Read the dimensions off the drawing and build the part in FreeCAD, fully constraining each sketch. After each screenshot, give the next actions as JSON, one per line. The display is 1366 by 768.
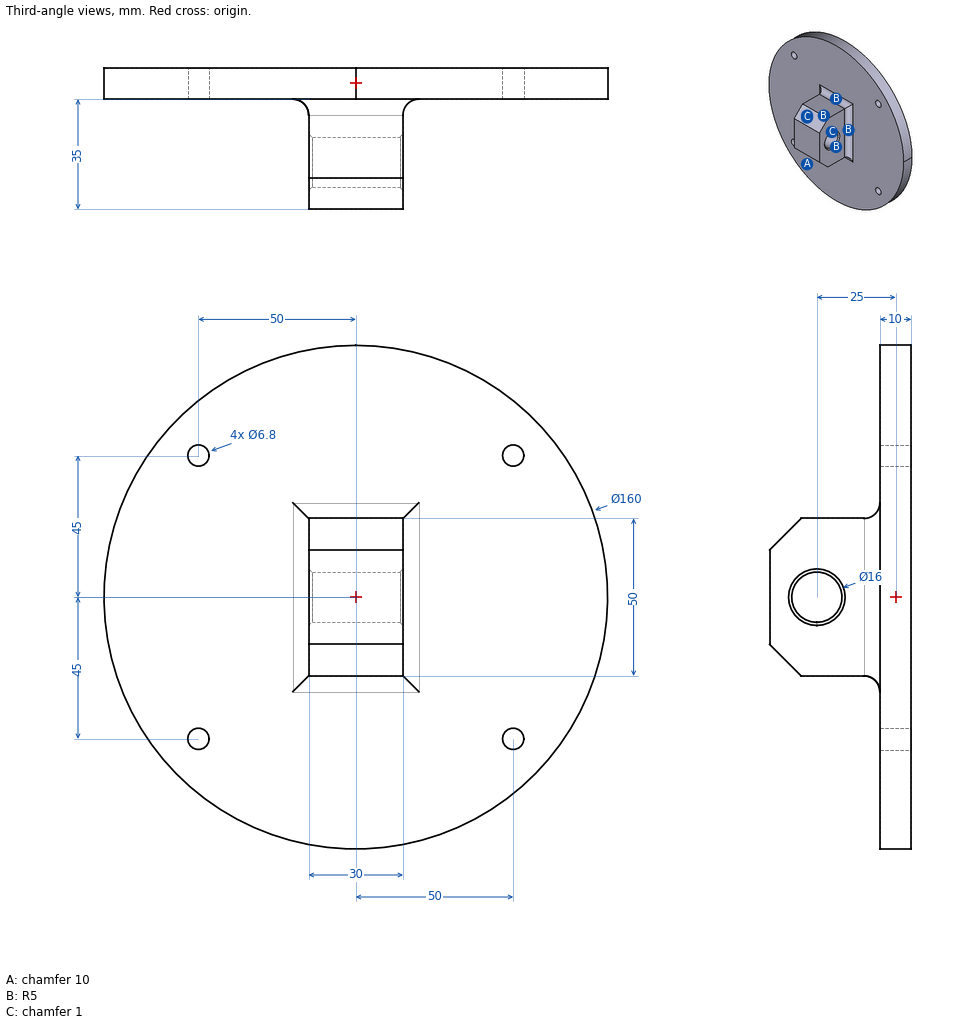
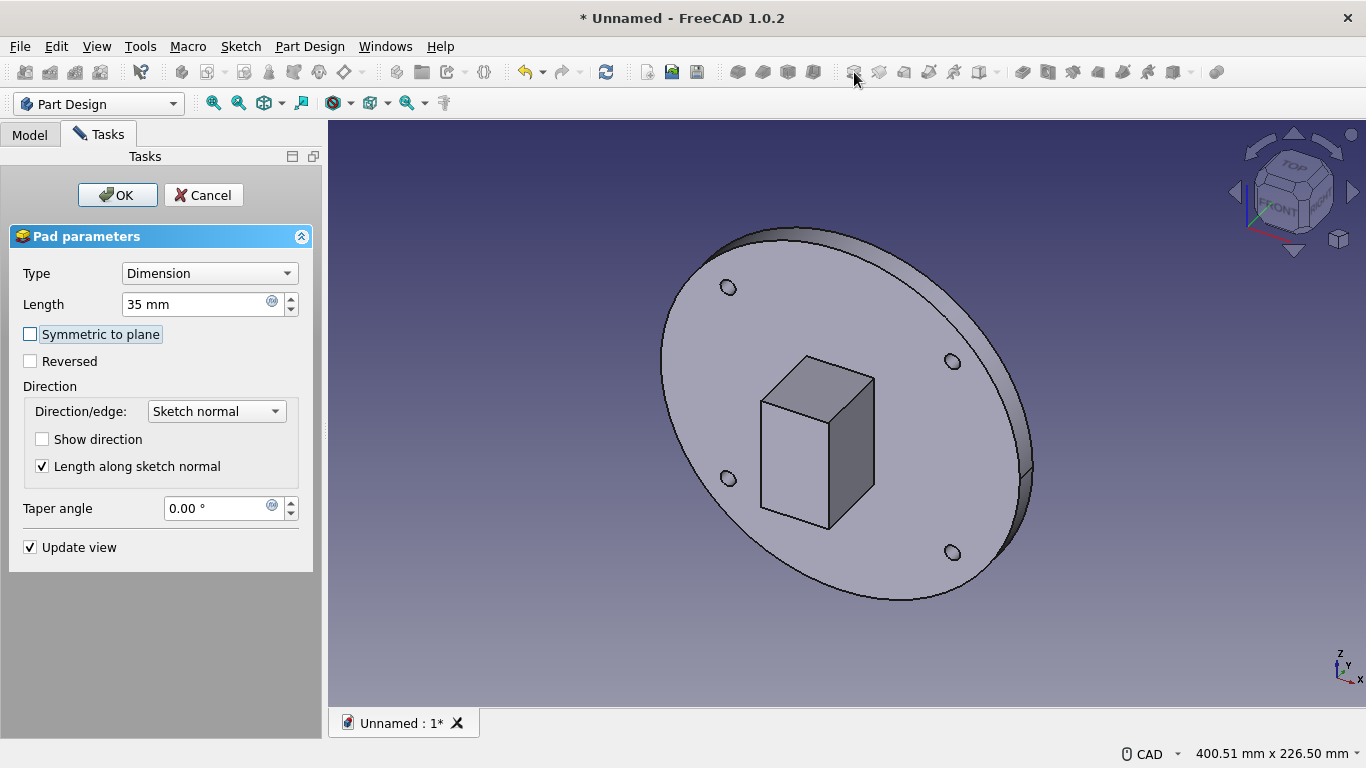
{"action": "left_click", "coordinate": [118, 195]}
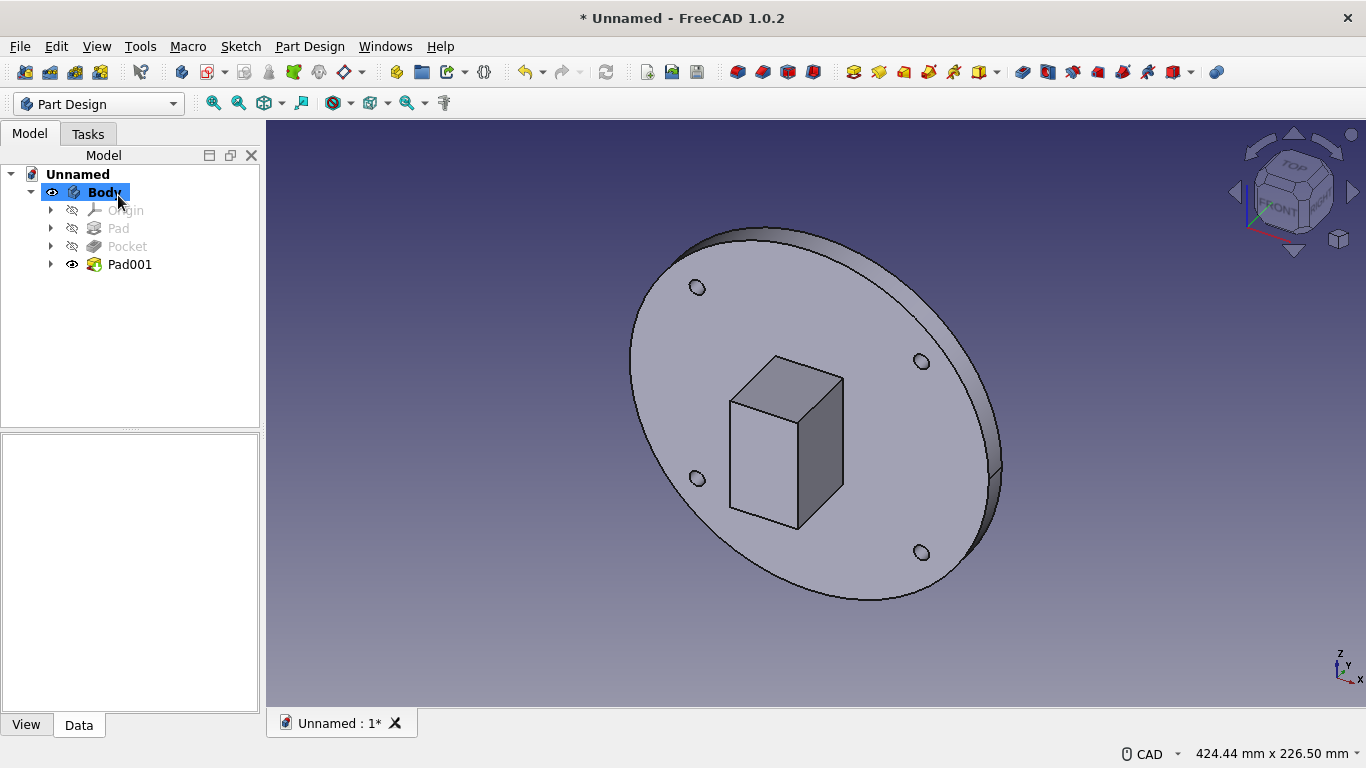
{"action": "left_click", "coordinate": [820, 438]}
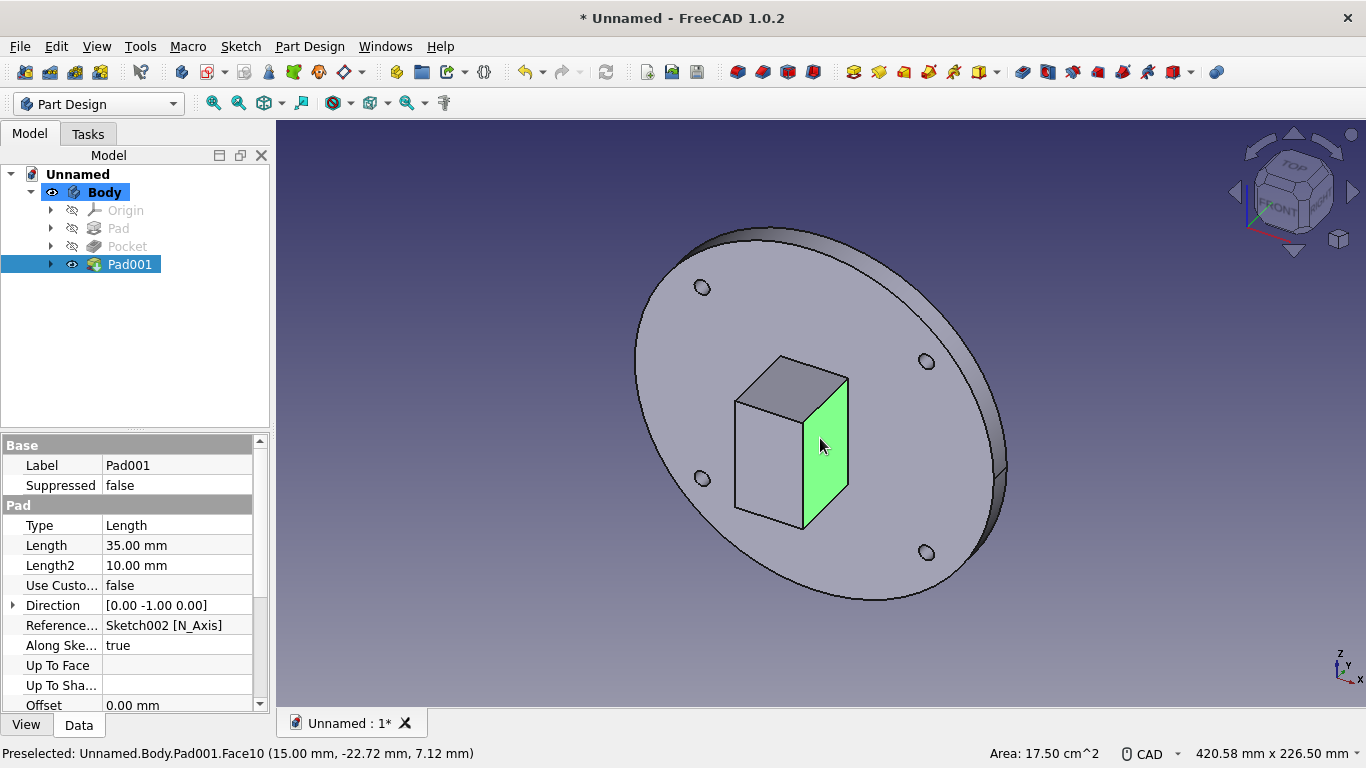
{"action": "left_click", "coordinate": [206, 72]}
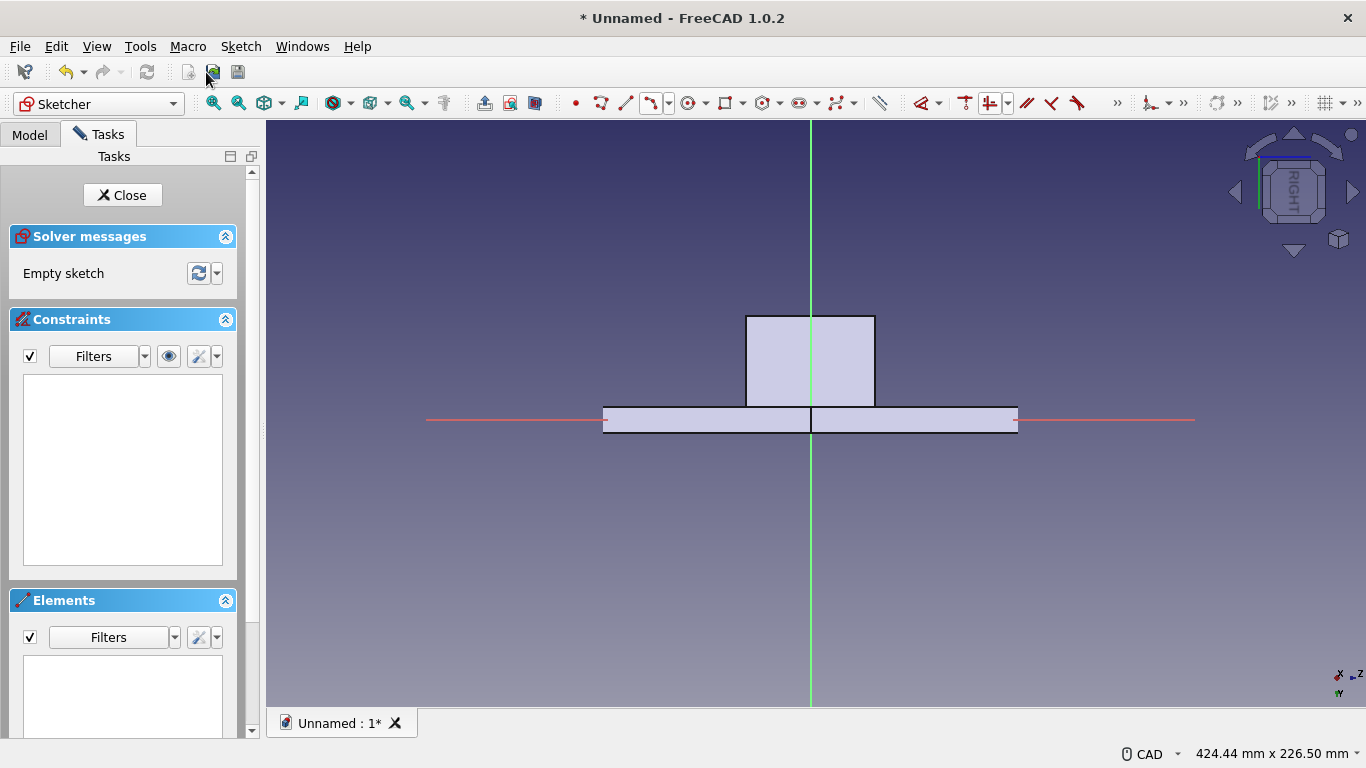
{"action": "left_click", "coordinate": [535, 104]}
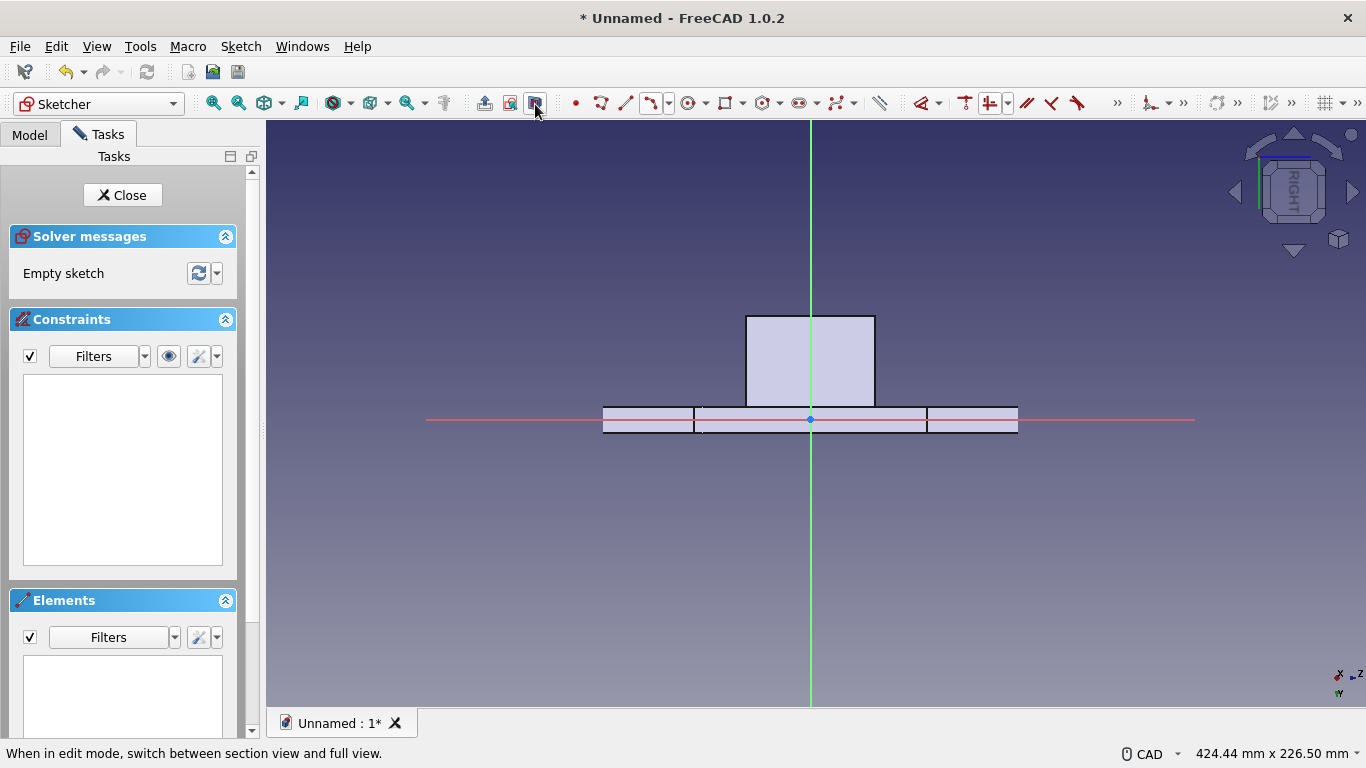
{"action": "scroll", "coordinate": [831, 365], "scroll_direction": "up", "scroll_amount": 7}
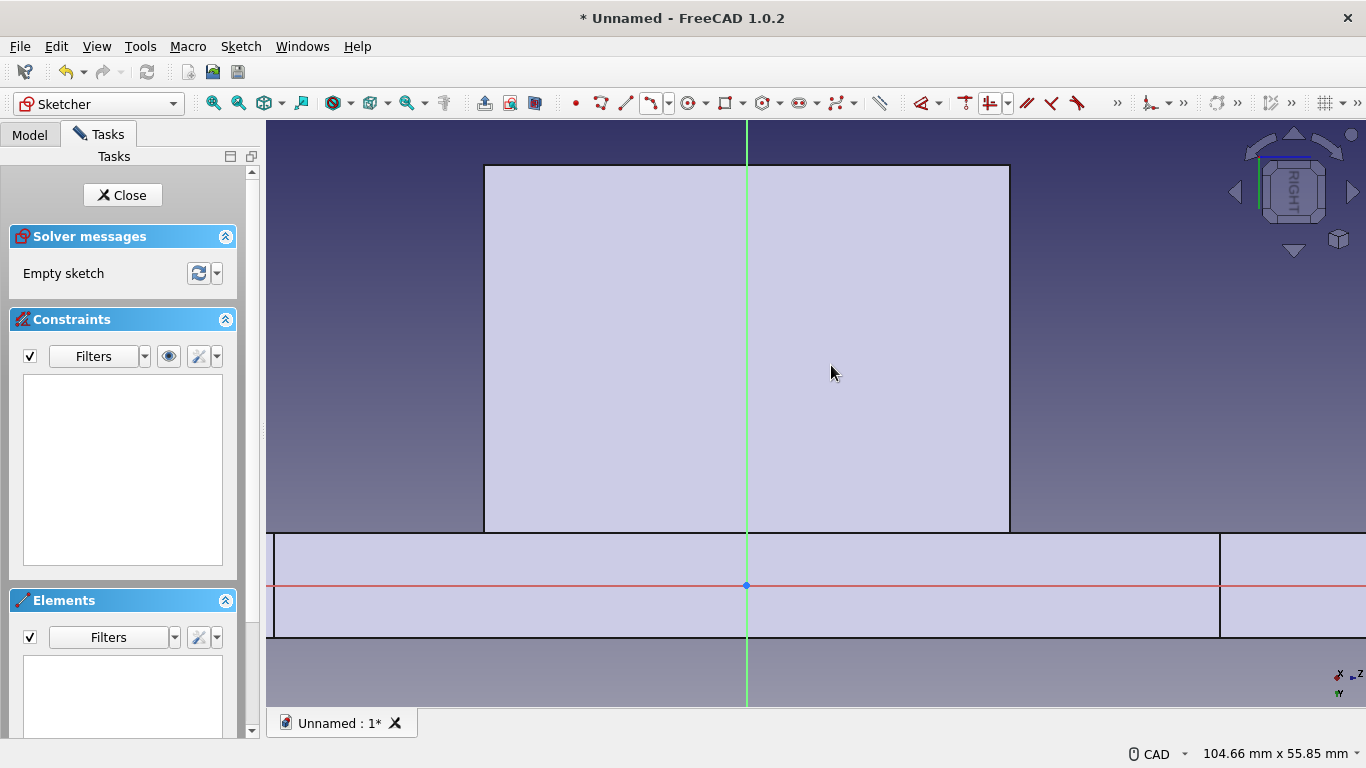
{"action": "key", "text": "g c"}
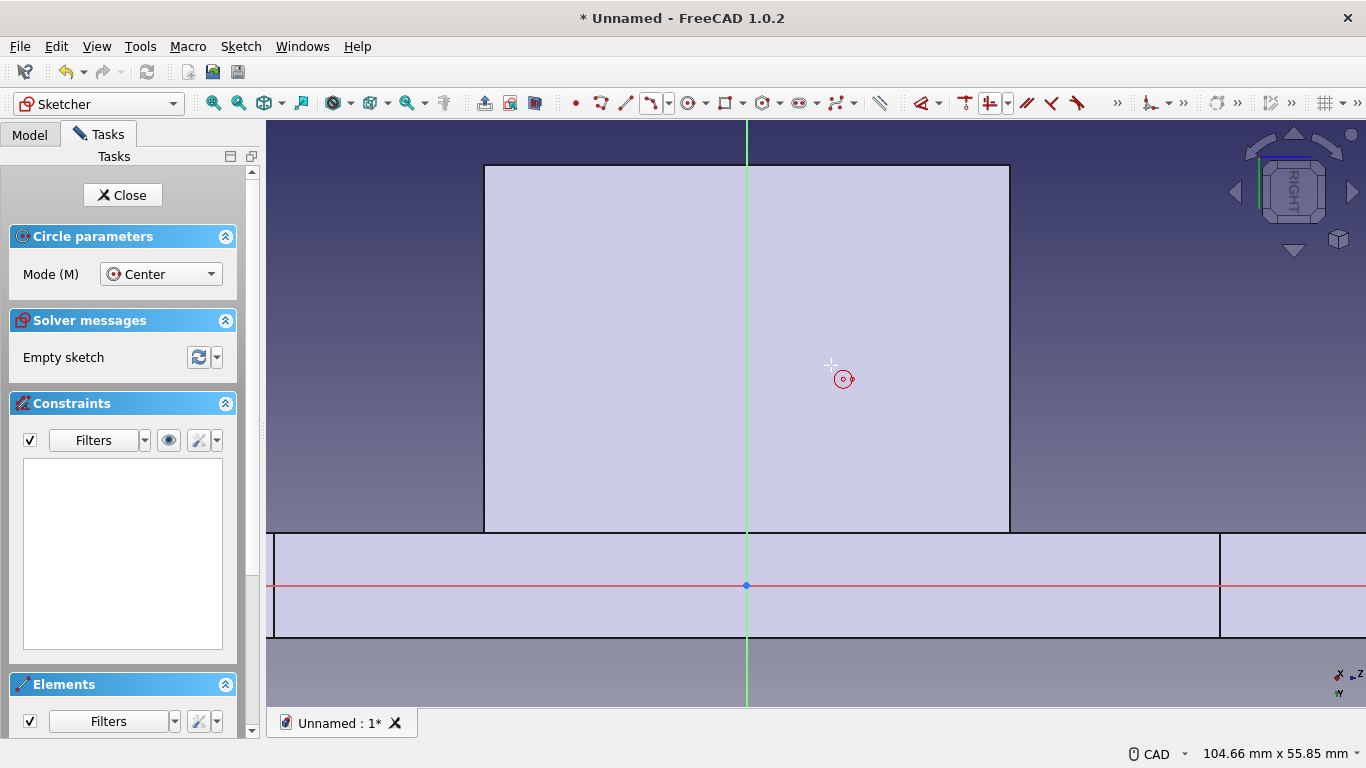
{"action": "left_click", "coordinate": [747, 323]}
{"action": "left_click", "coordinate": [806, 263]}
{"action": "key", "text": "Escape"}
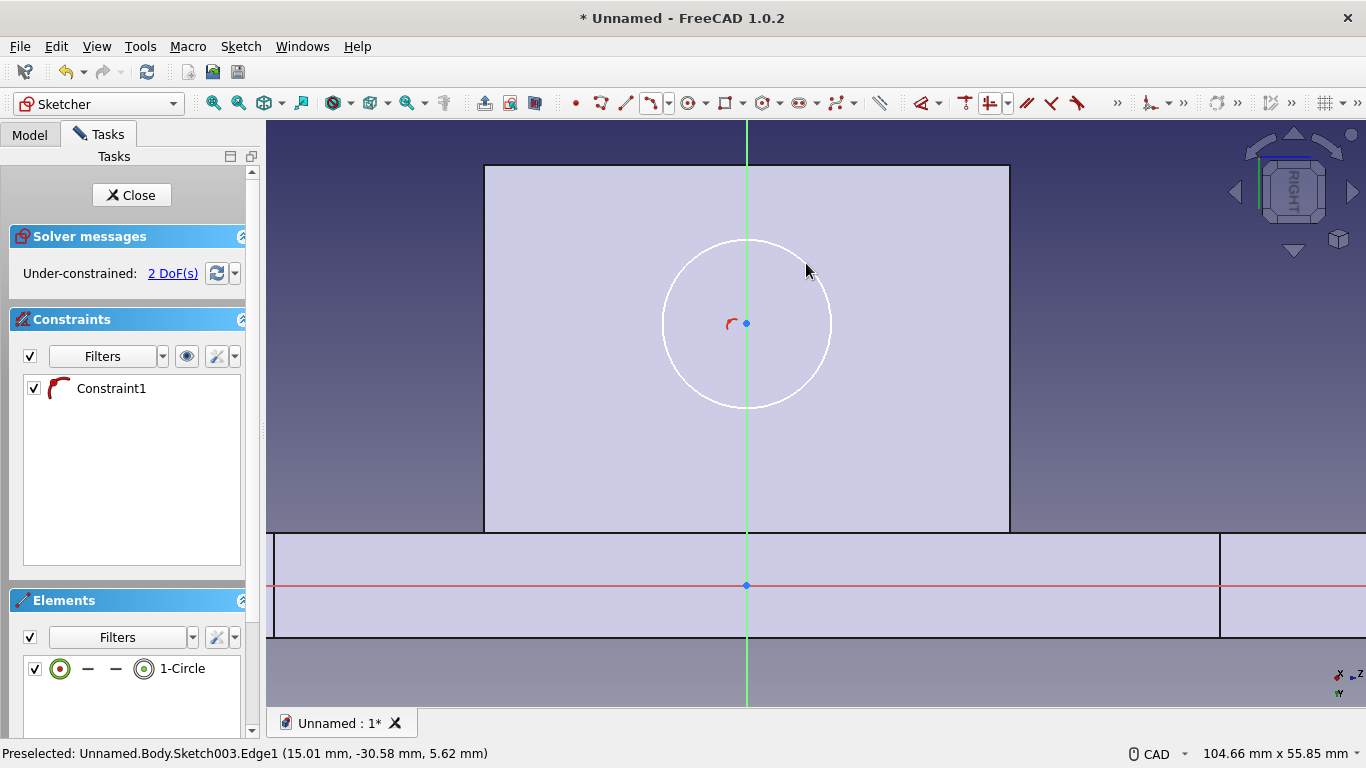
{"action": "key", "text": "d"}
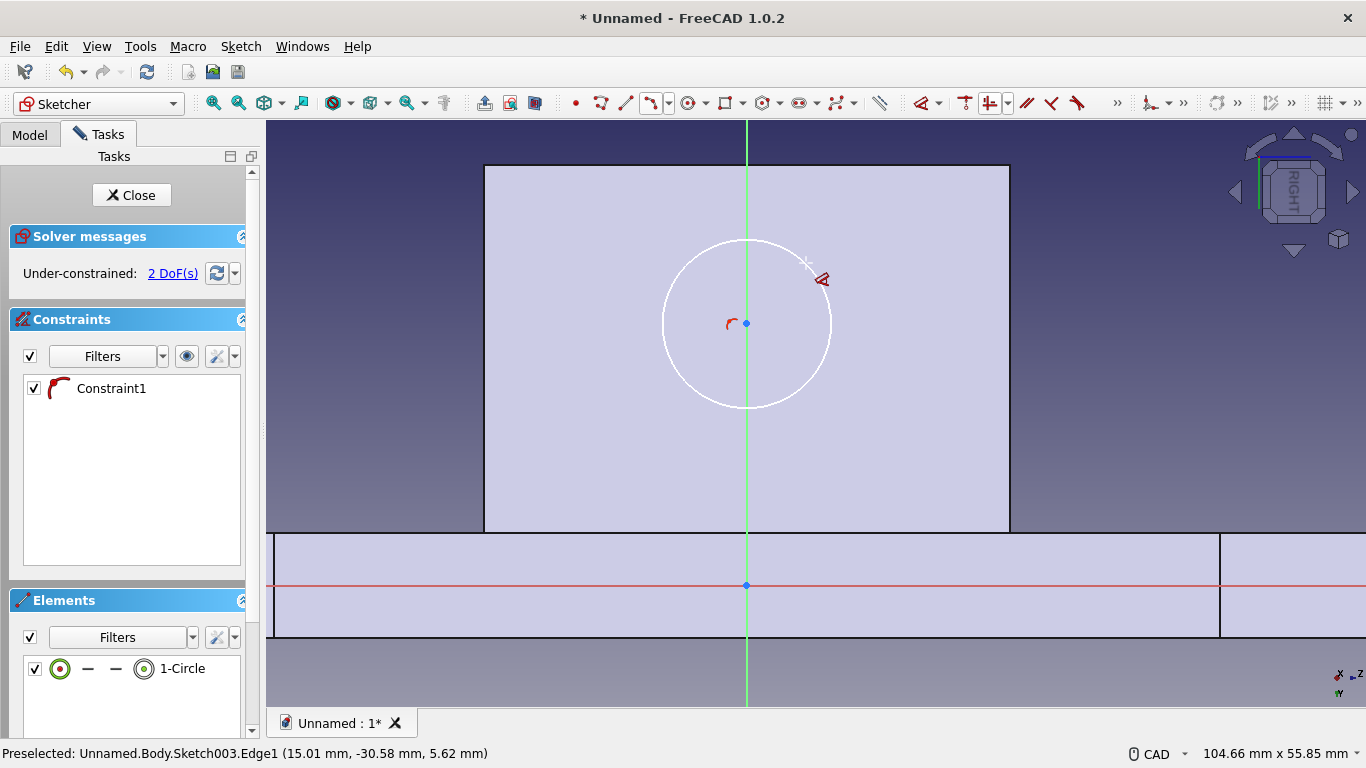
{"action": "left_click", "coordinate": [806, 264]}
{"action": "left_click", "coordinate": [828, 241]}